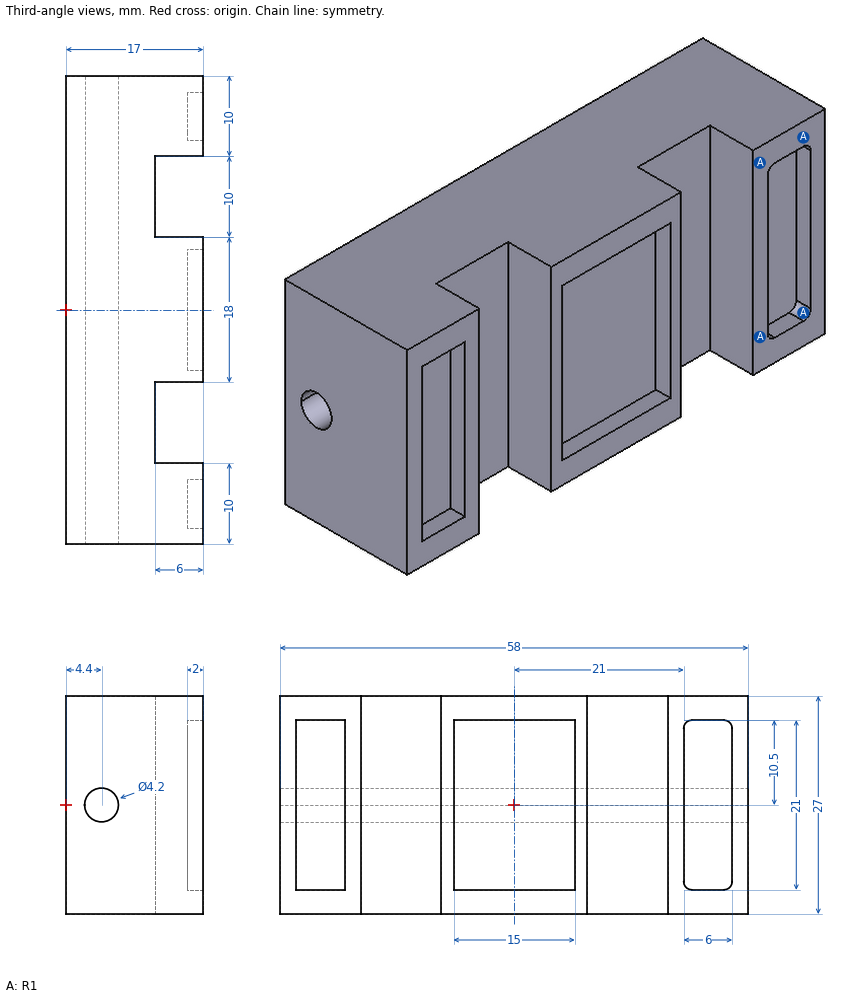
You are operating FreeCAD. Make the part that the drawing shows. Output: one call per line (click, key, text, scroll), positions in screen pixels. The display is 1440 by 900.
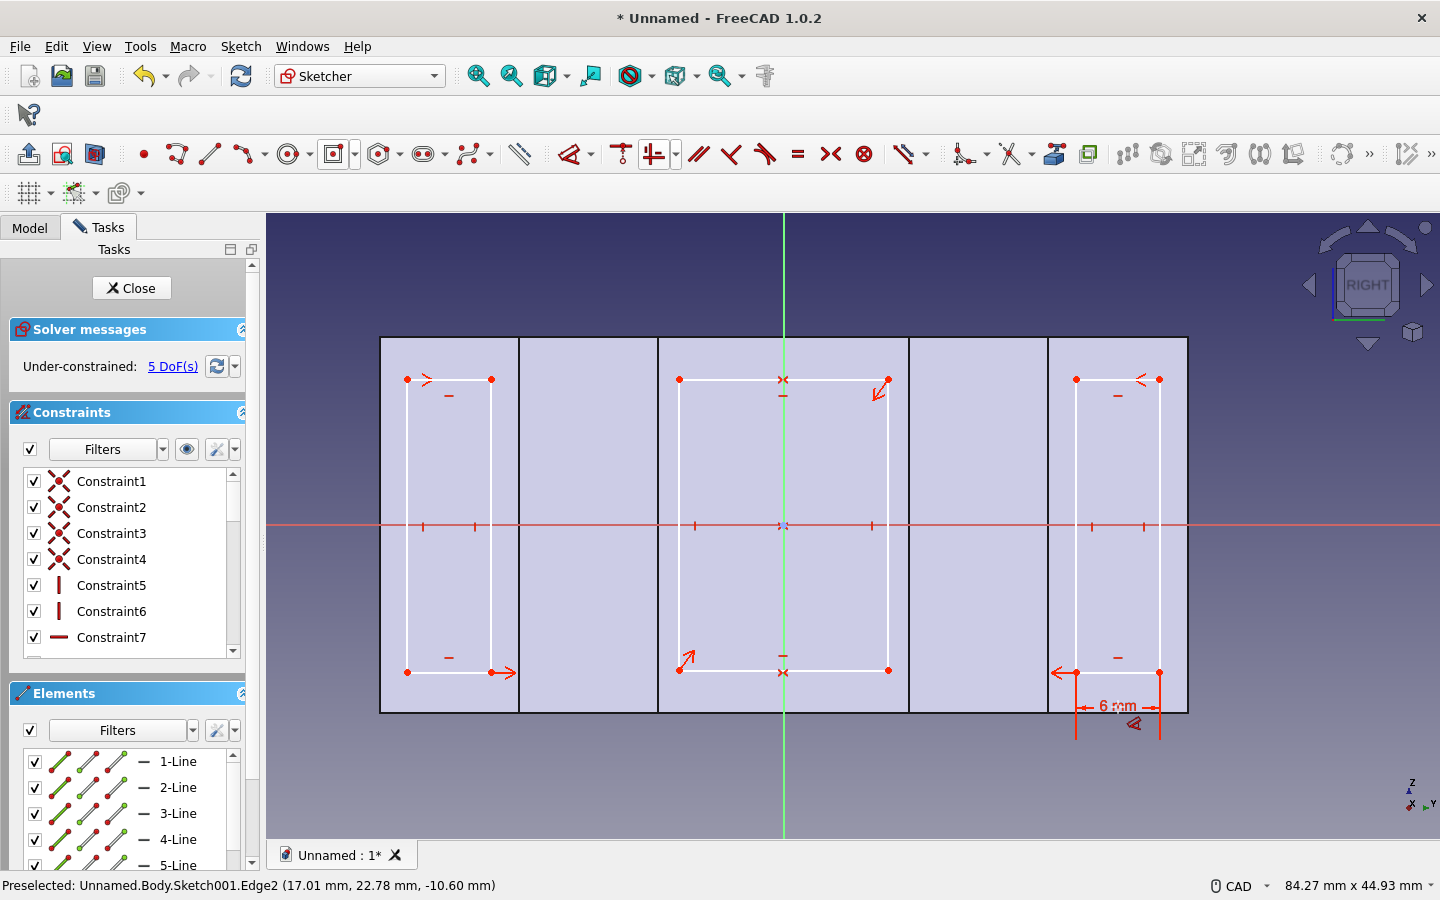
click(1076, 468)
click(1110, 459)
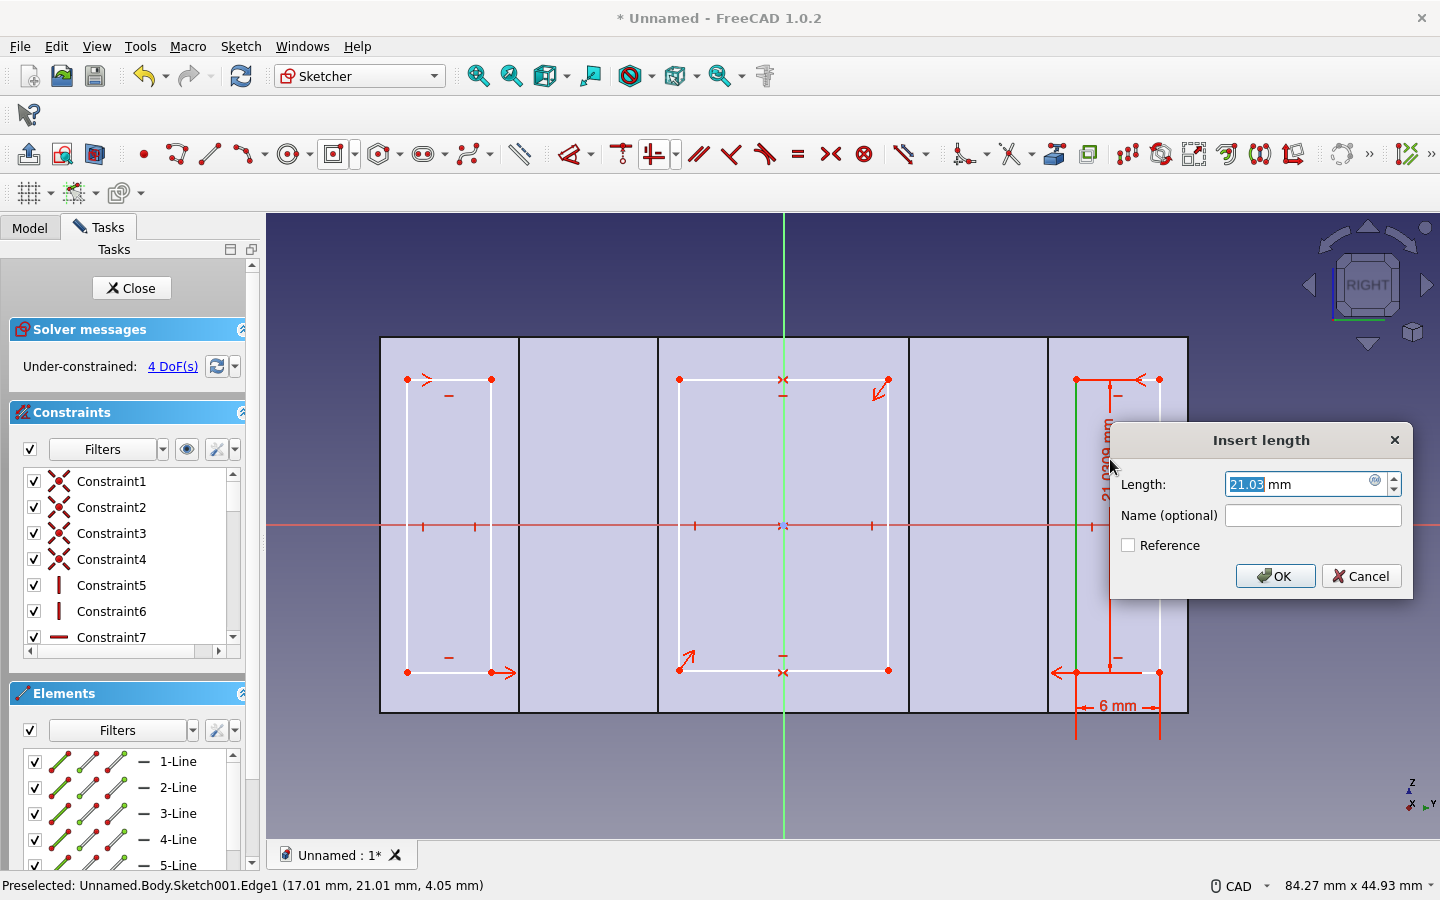
text(21)
key(Return)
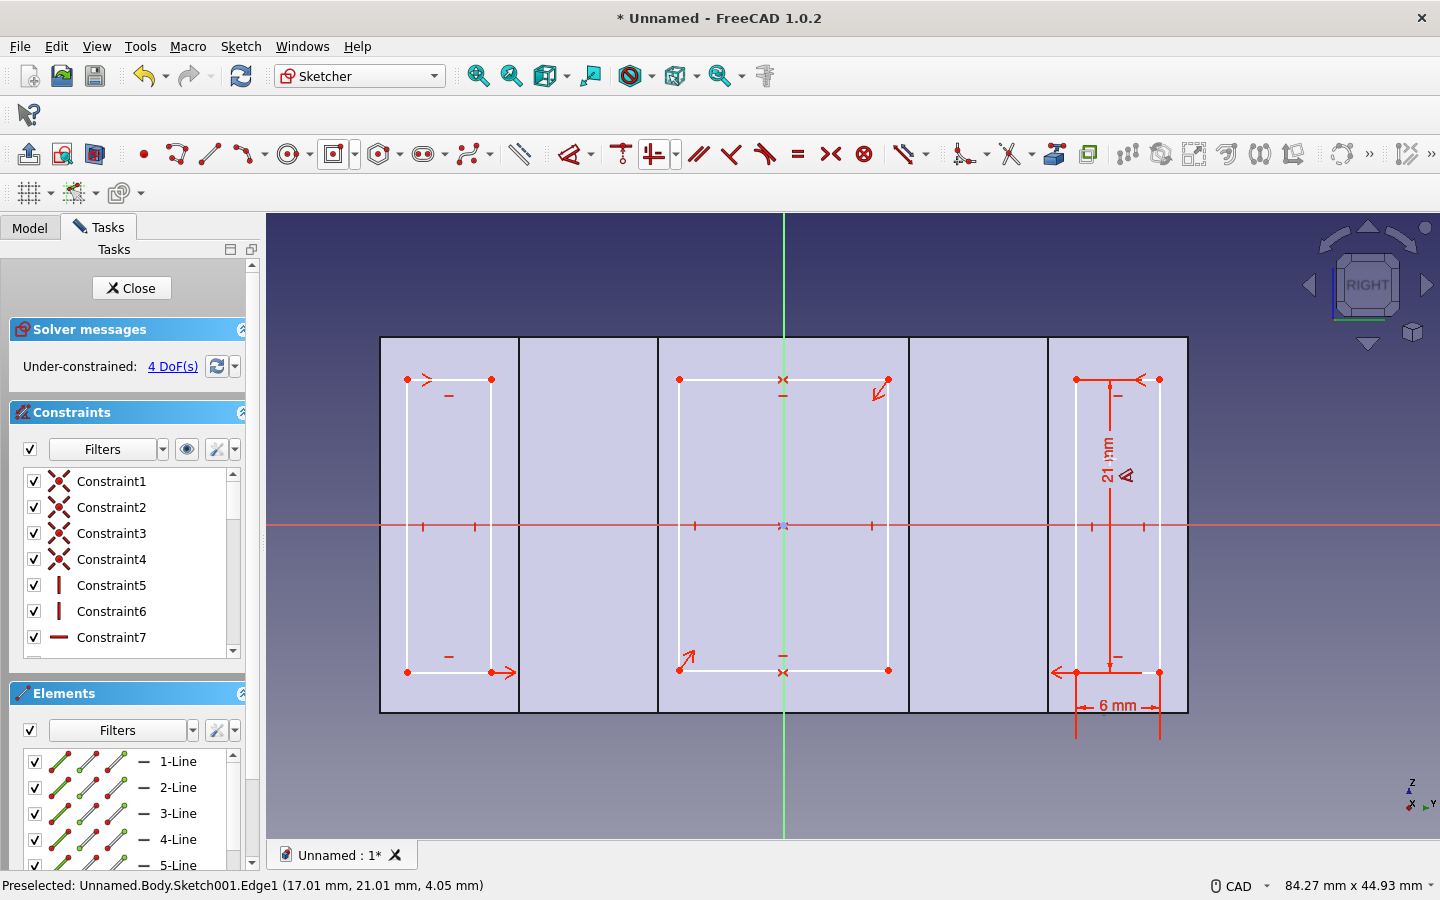
click(742, 671)
click(736, 705)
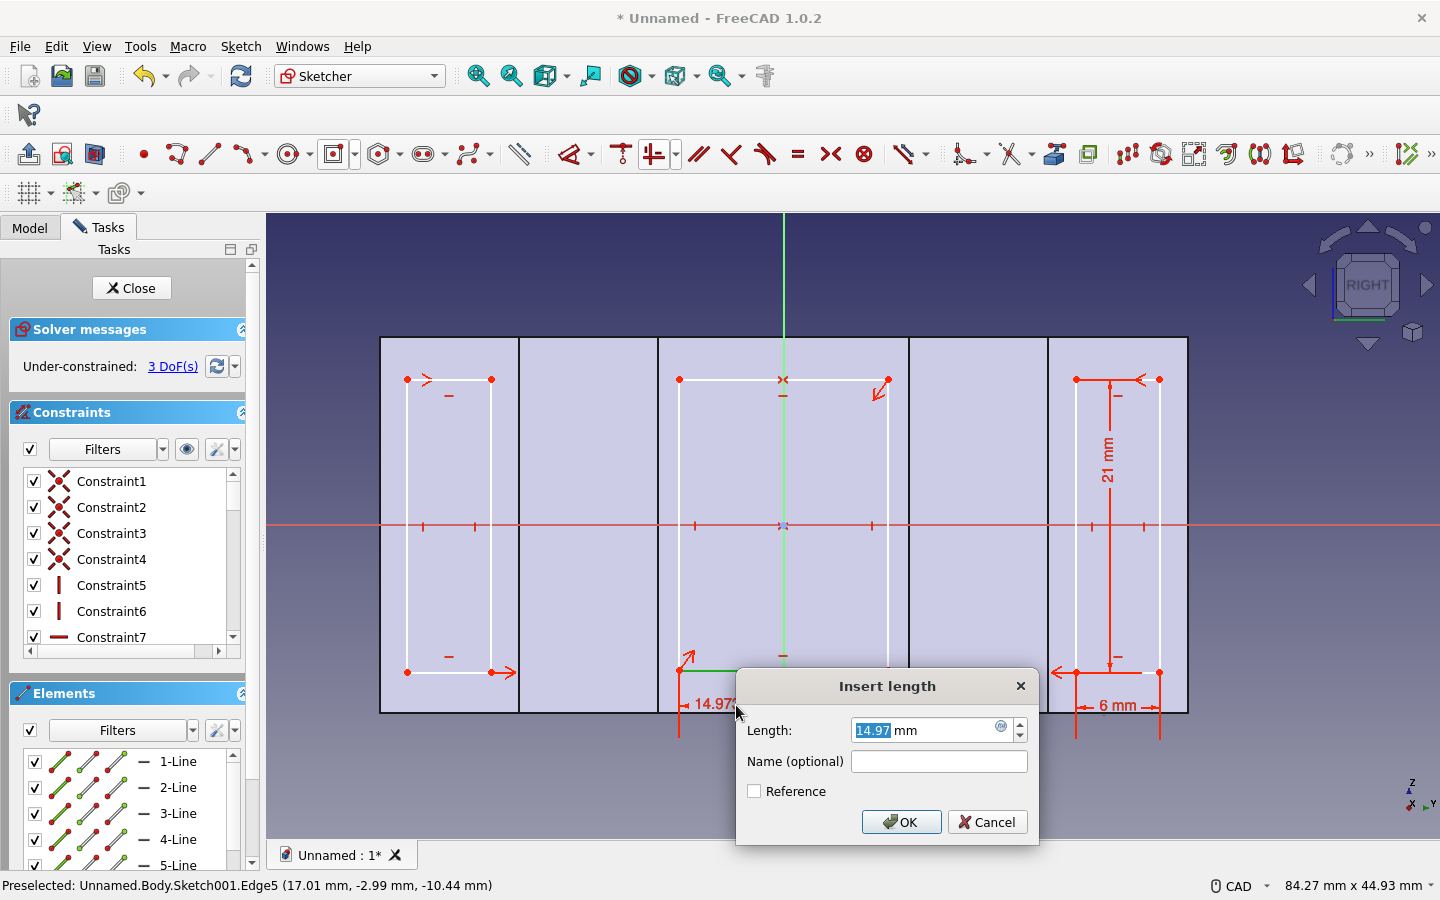
text(15)
key(Return)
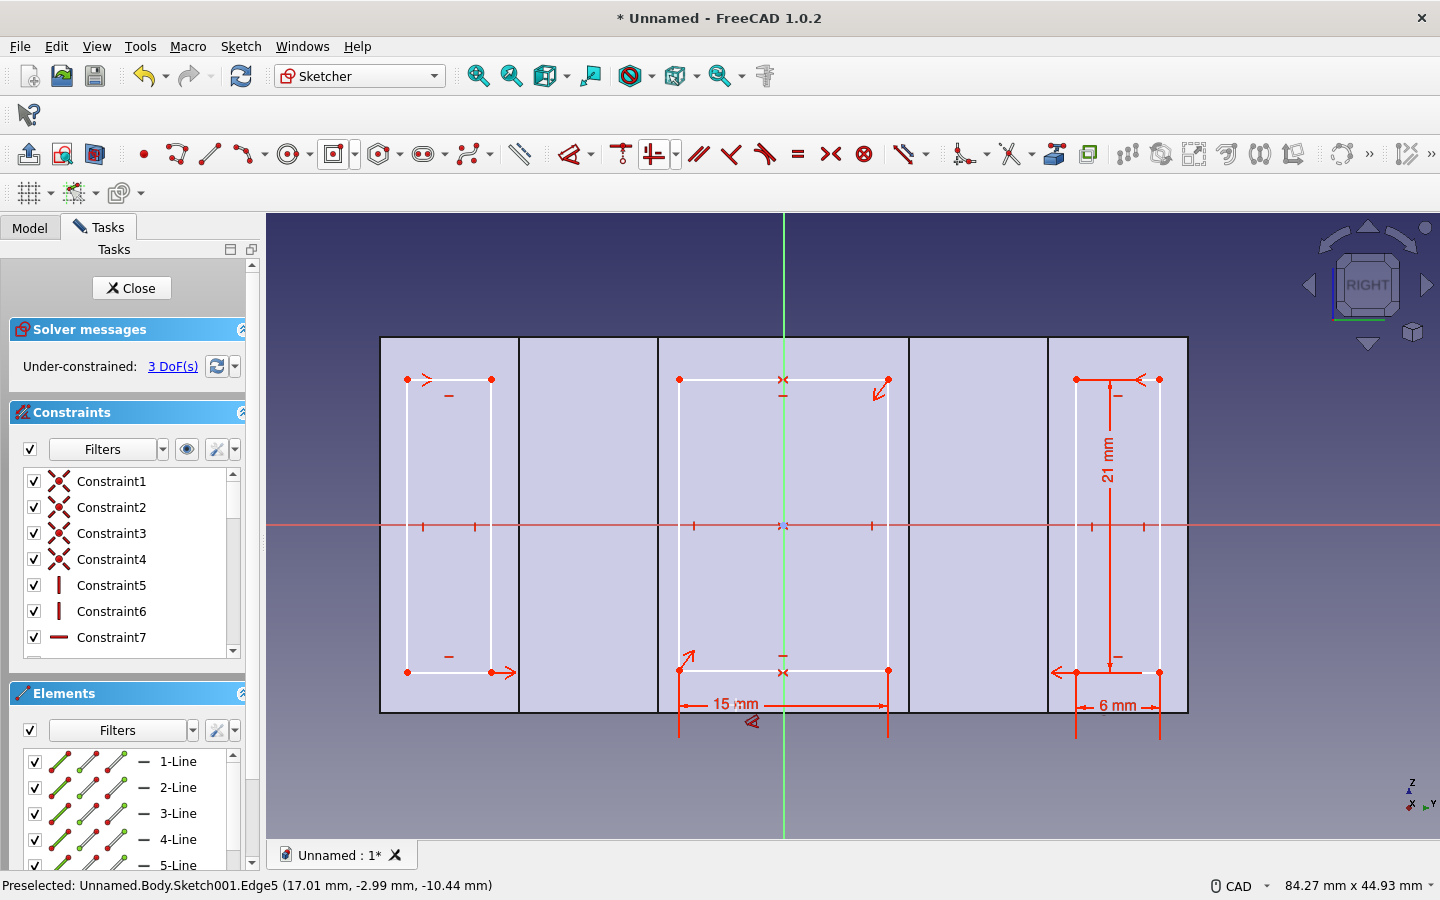
click(888, 584)
click(922, 459)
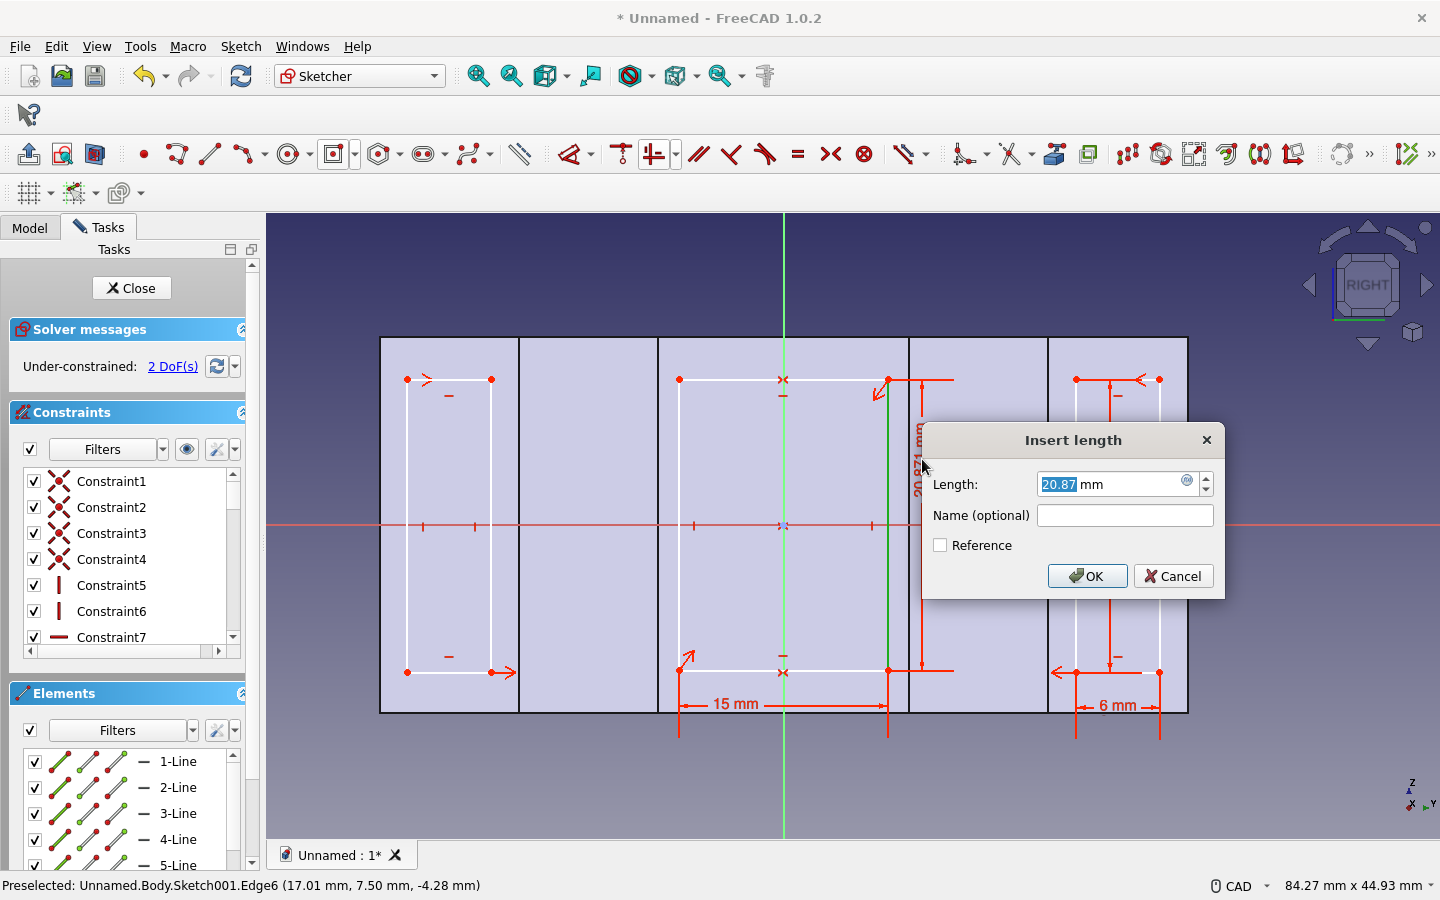
text(21)
key(Return)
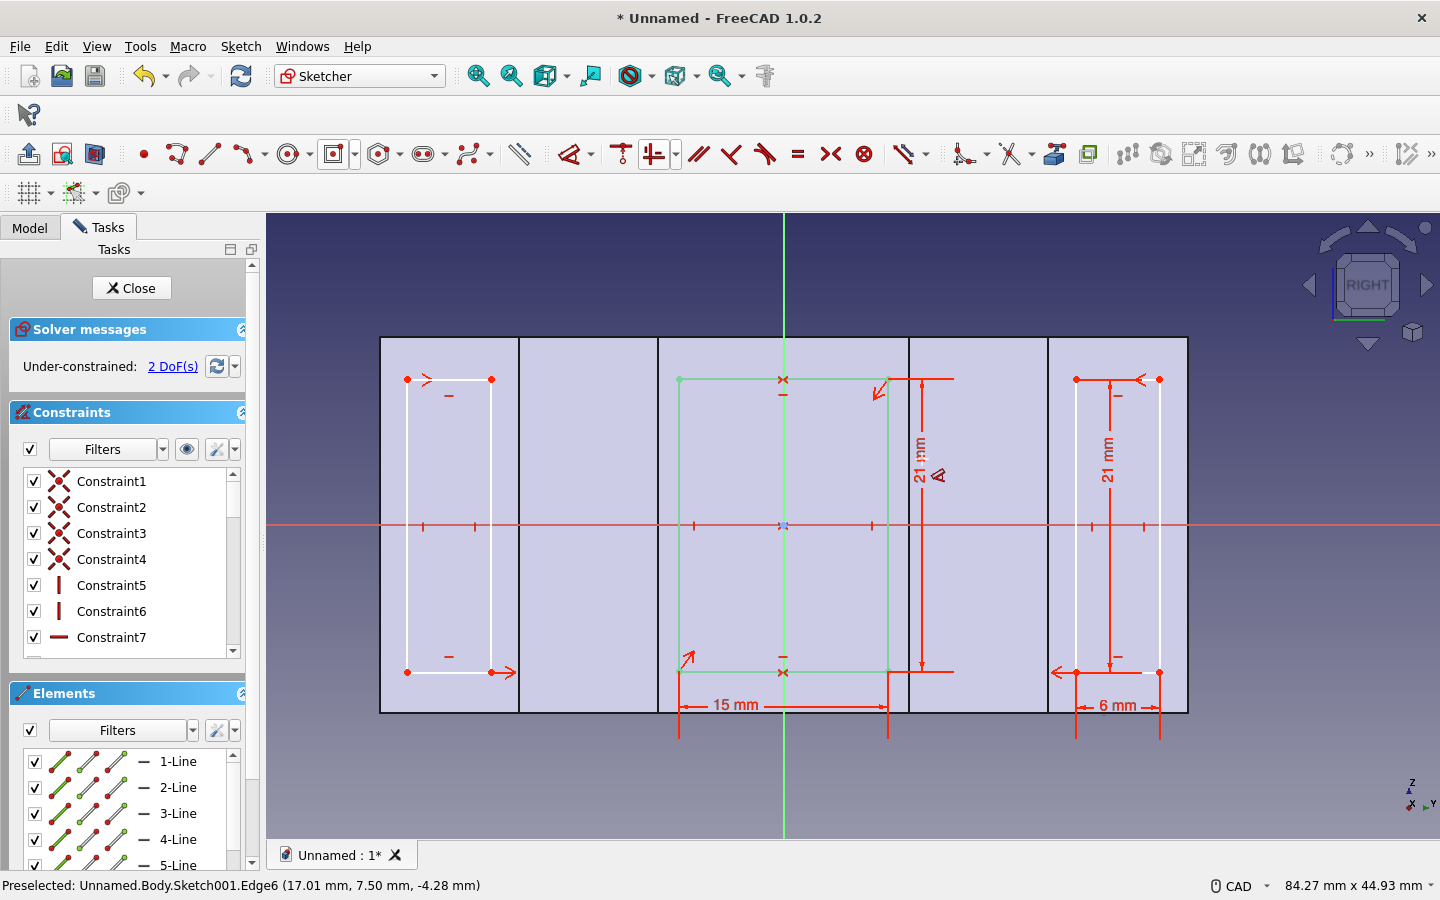
click(1076, 380)
click(930, 346)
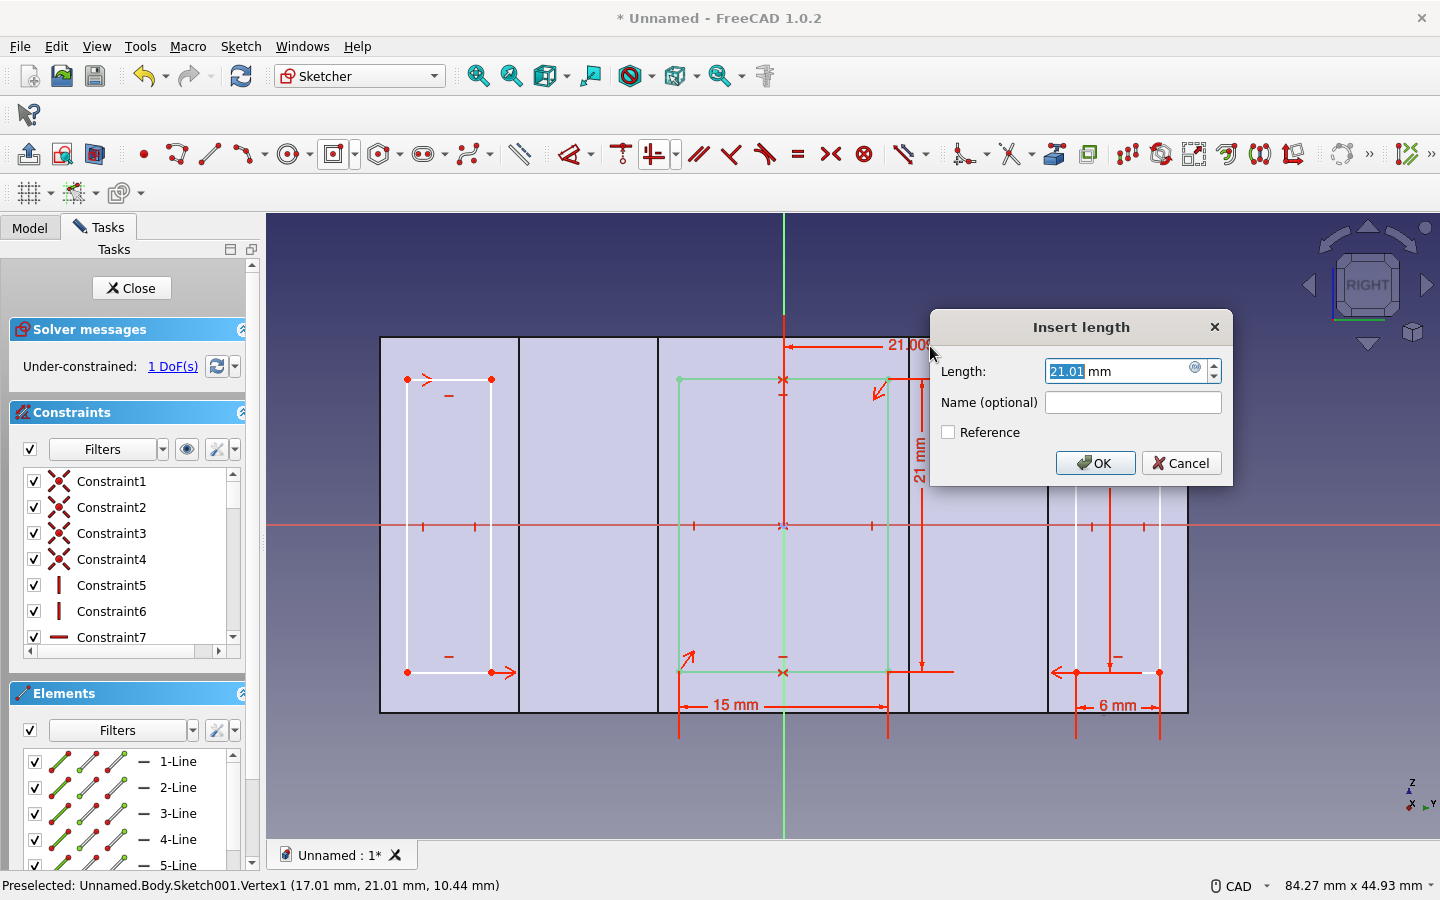
text(21)
key(Return)